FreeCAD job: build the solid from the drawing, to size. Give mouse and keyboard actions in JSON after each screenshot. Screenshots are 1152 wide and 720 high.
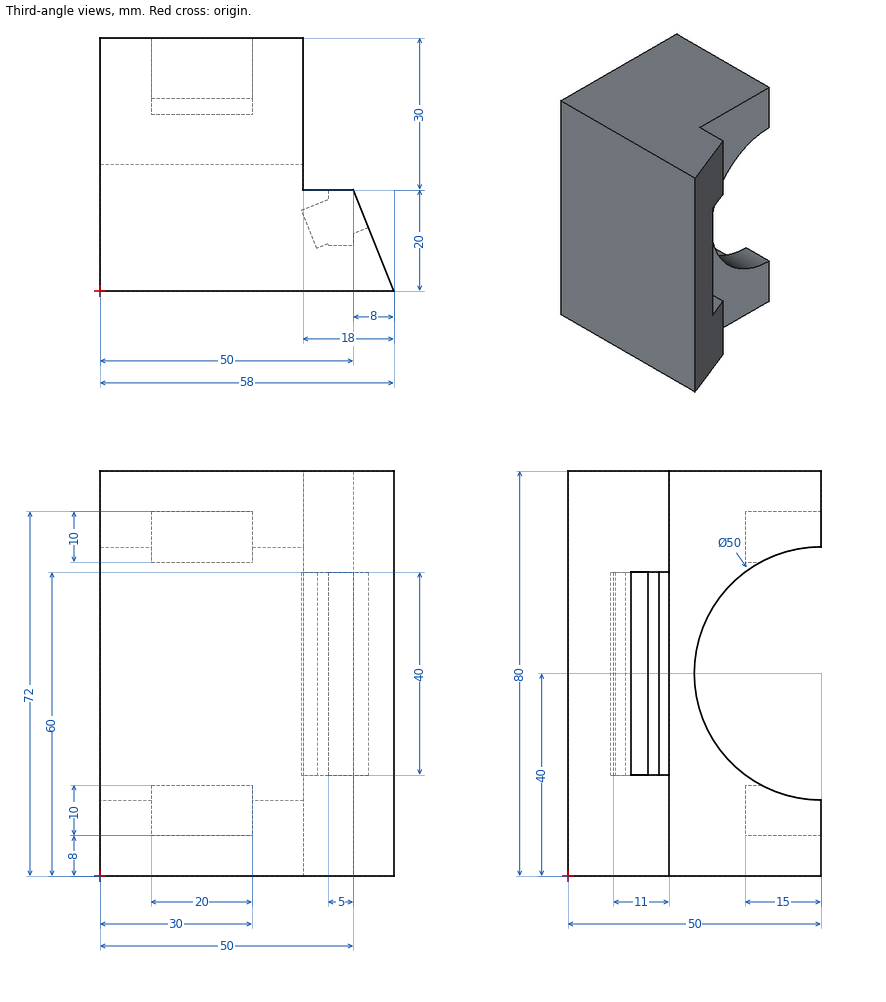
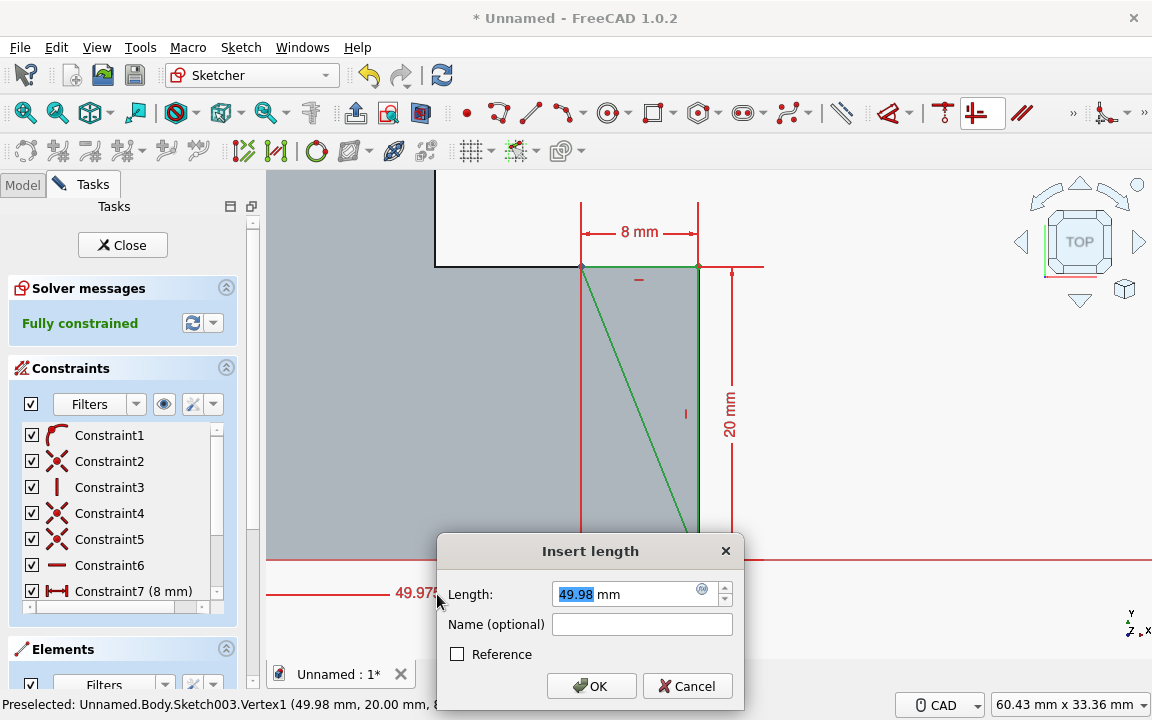
{"action": "type", "text": "50"}
{"action": "key", "text": "Return"}
{"action": "key", "text": "Escape"}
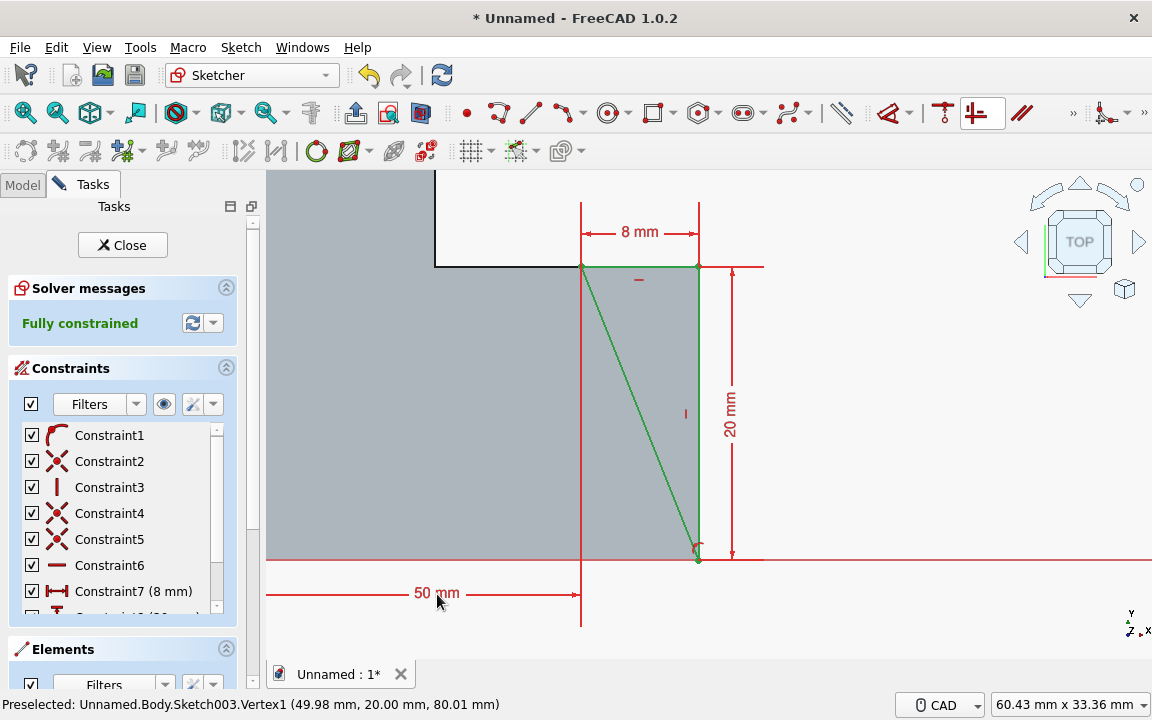
{"action": "left_click", "coordinate": [123, 245]}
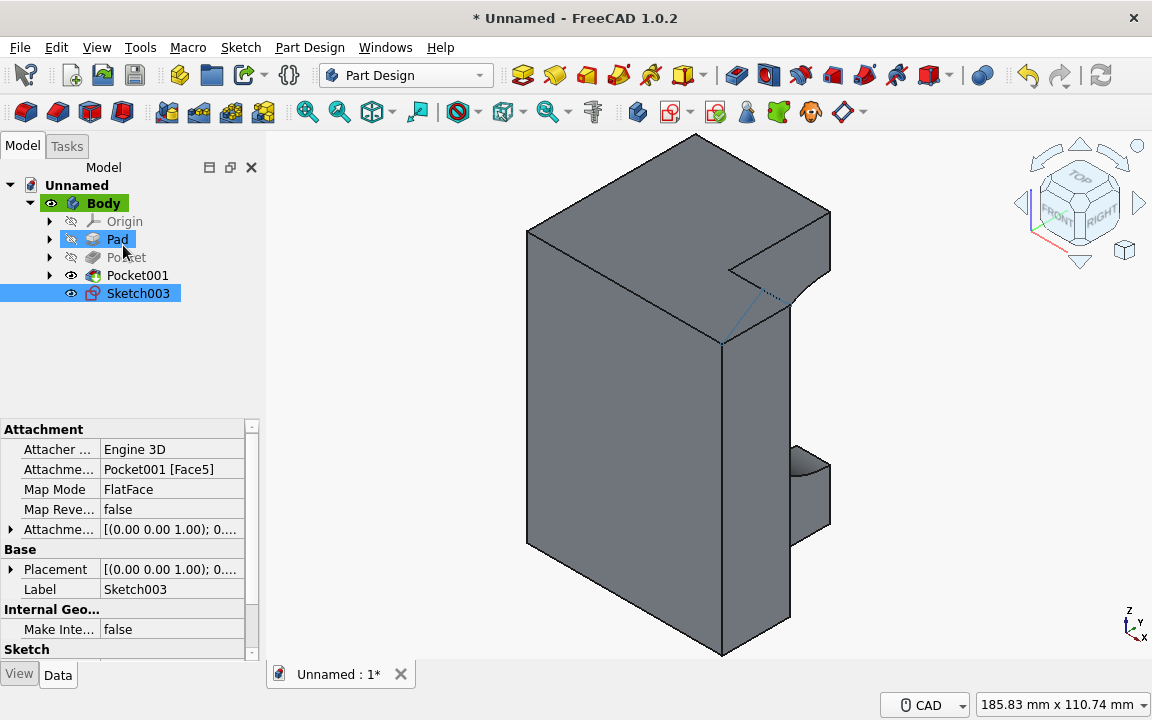
{"action": "left_click", "coordinate": [738, 76]}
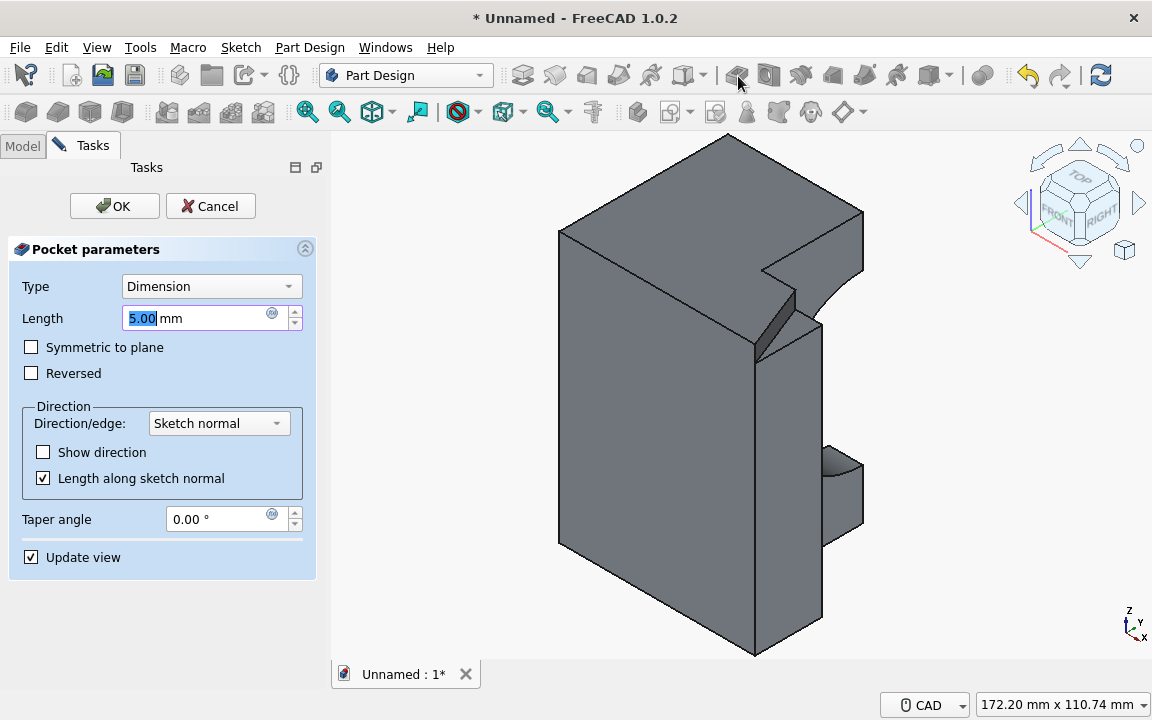
{"action": "left_click", "coordinate": [212, 286]}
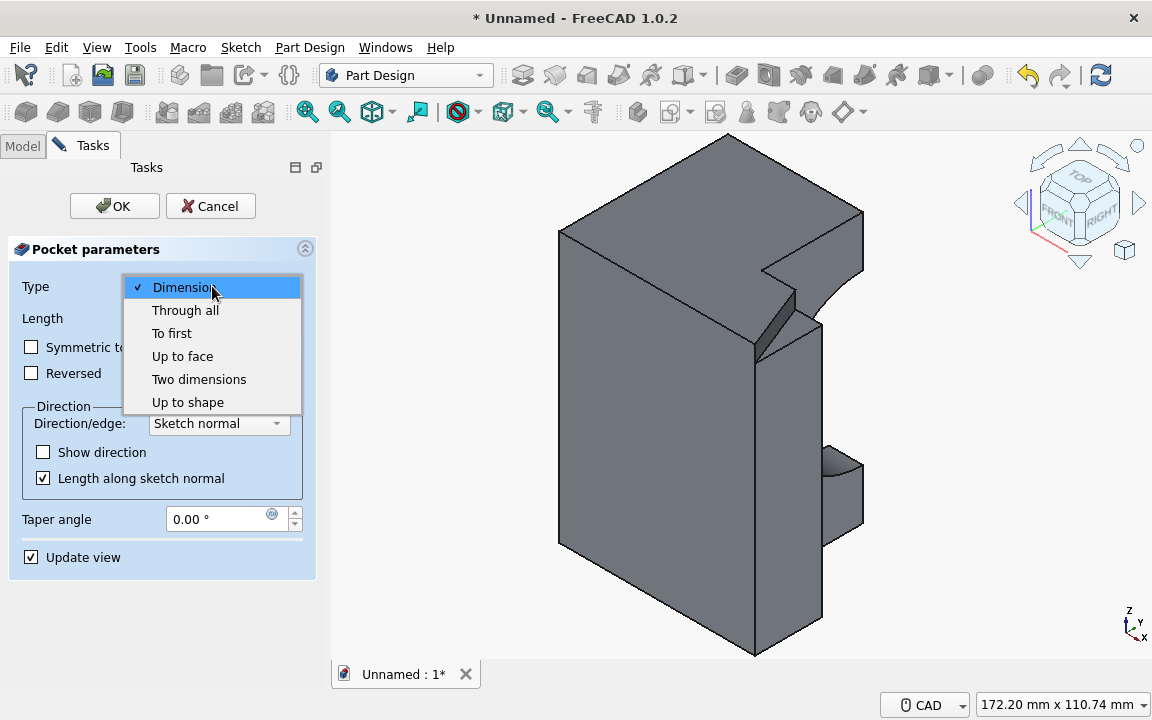
{"action": "left_click", "coordinate": [212, 310]}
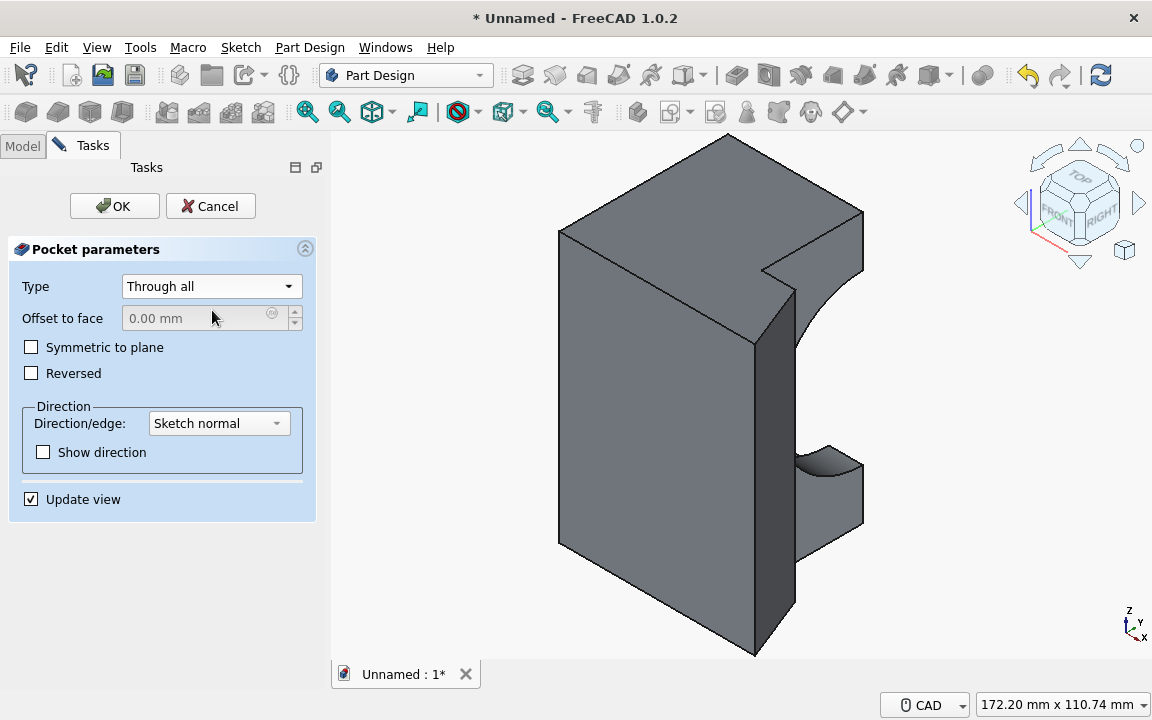
{"action": "left_click", "coordinate": [115, 206]}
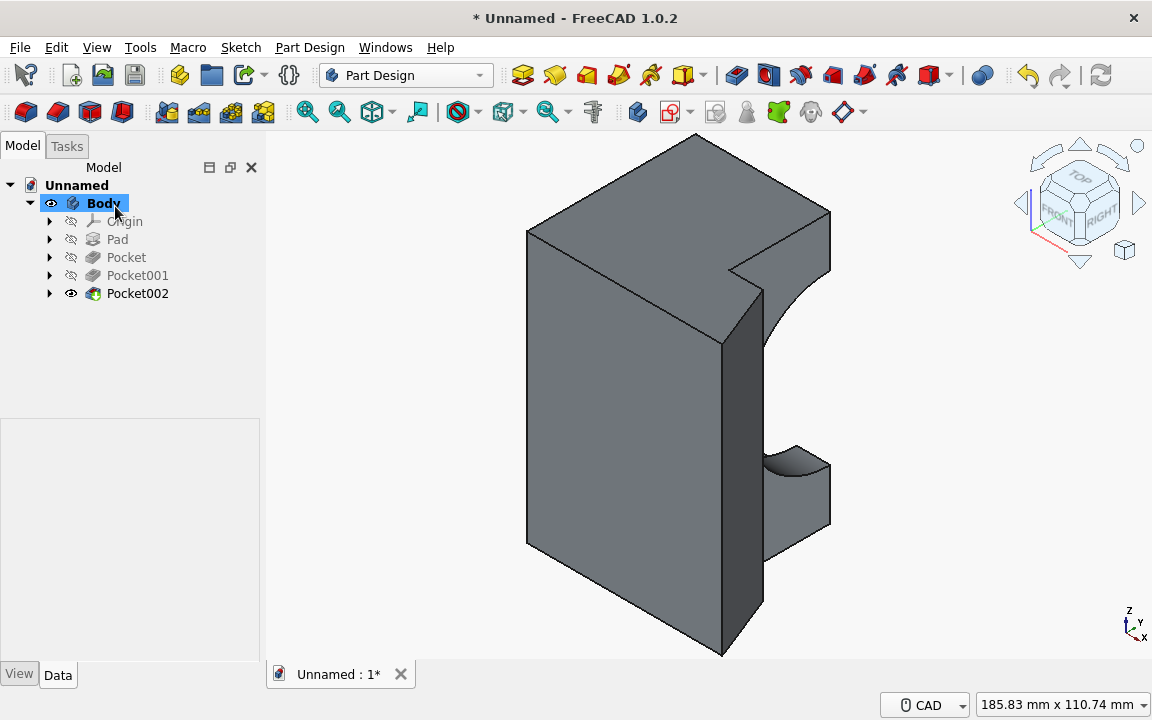
{"action": "key", "text": "4"}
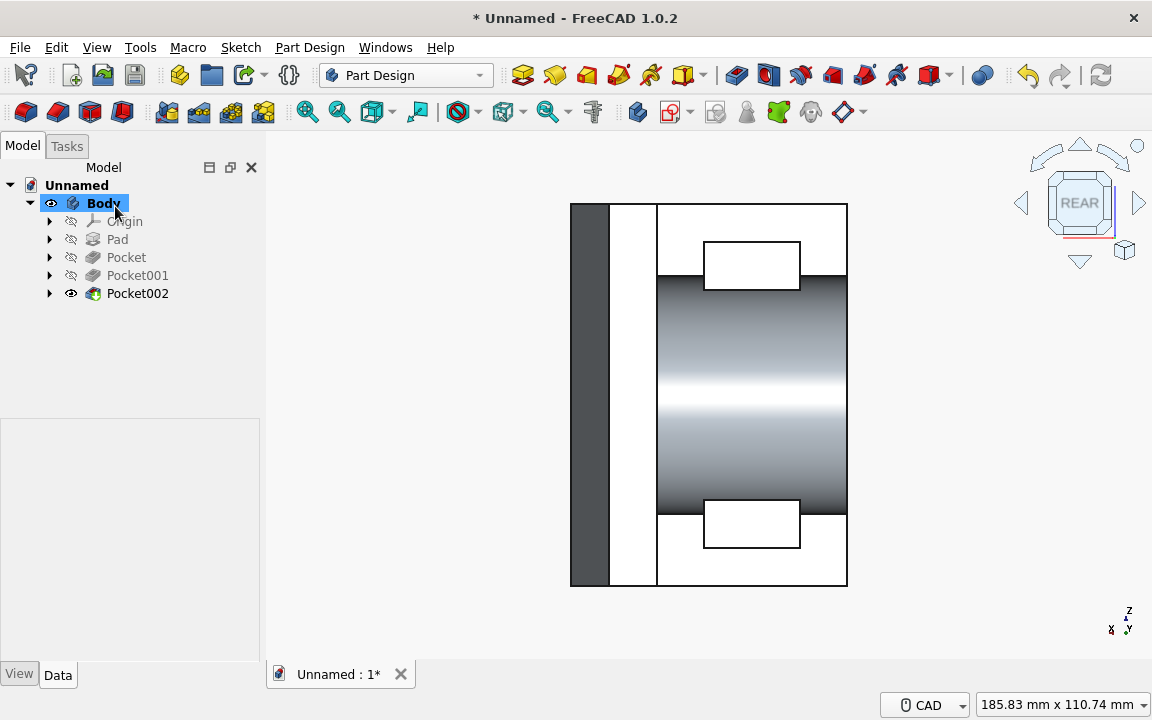
{"action": "left_click", "coordinate": [633, 231]}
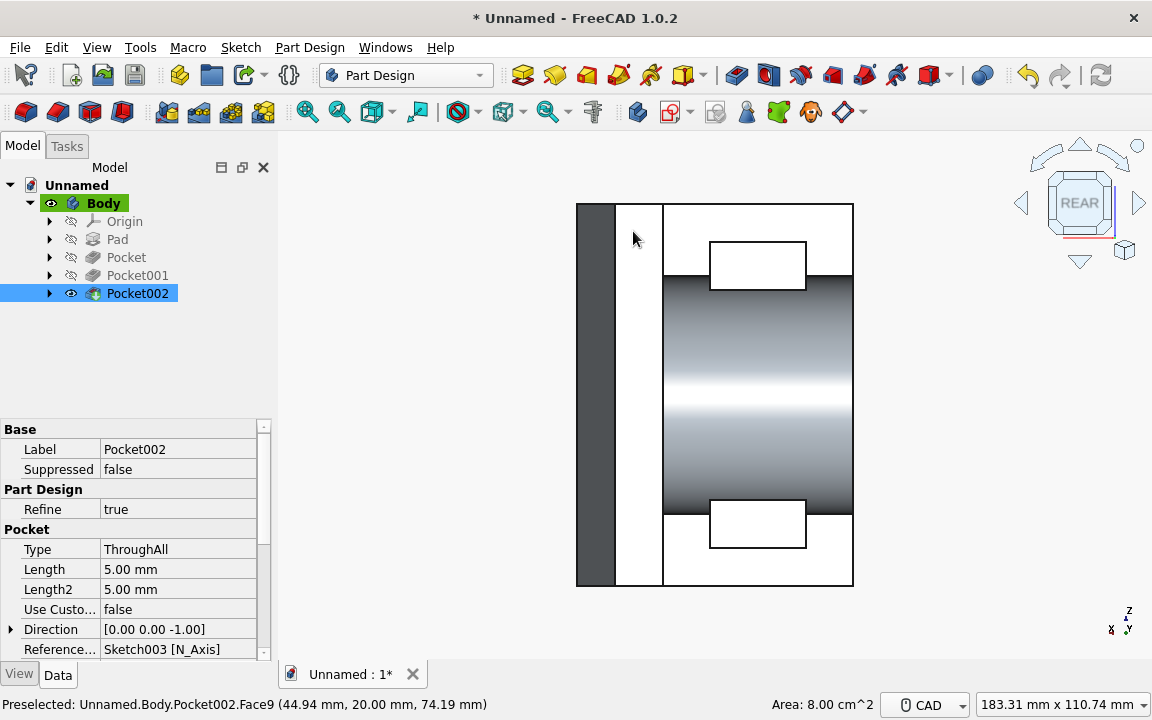
{"action": "left_click", "coordinate": [670, 112]}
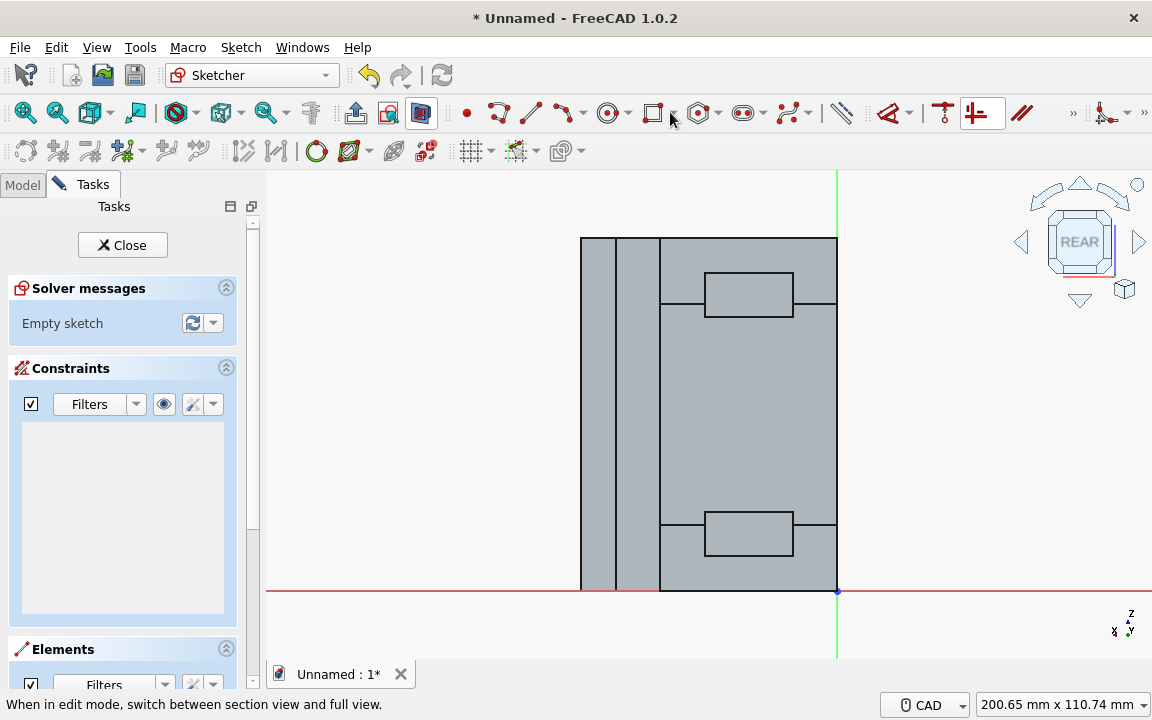
{"action": "left_click", "coordinate": [654, 114]}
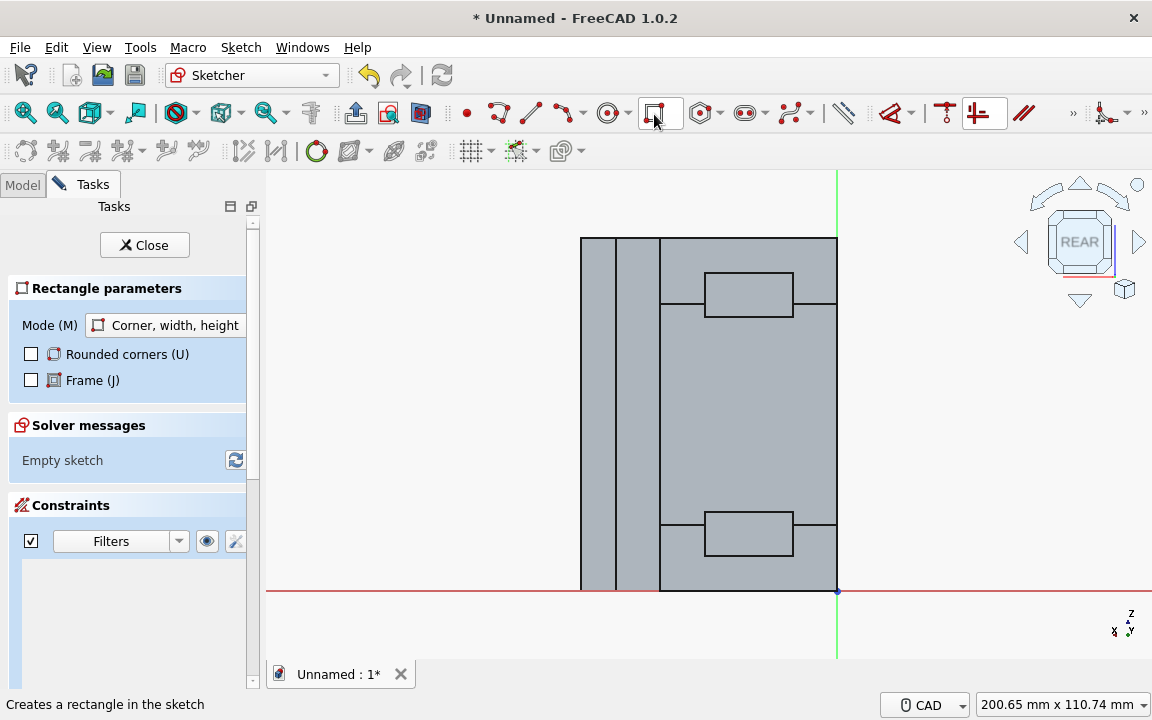
{"action": "left_click", "coordinate": [616, 326]}
{"action": "mouse_move", "coordinate": [638, 503]}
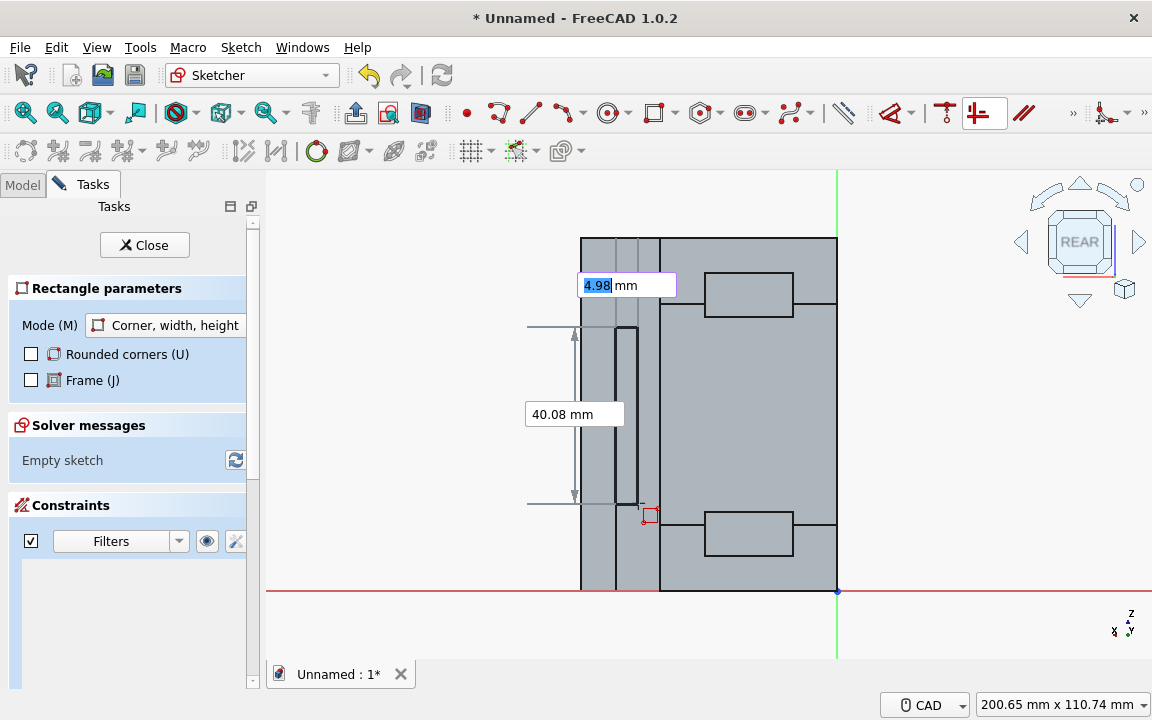
{"action": "type", "text": "5"}
{"action": "key", "text": "Tab"}
{"action": "type", "text": "40"}
{"action": "key", "text": "Return"}
{"action": "key", "text": "Escape"}